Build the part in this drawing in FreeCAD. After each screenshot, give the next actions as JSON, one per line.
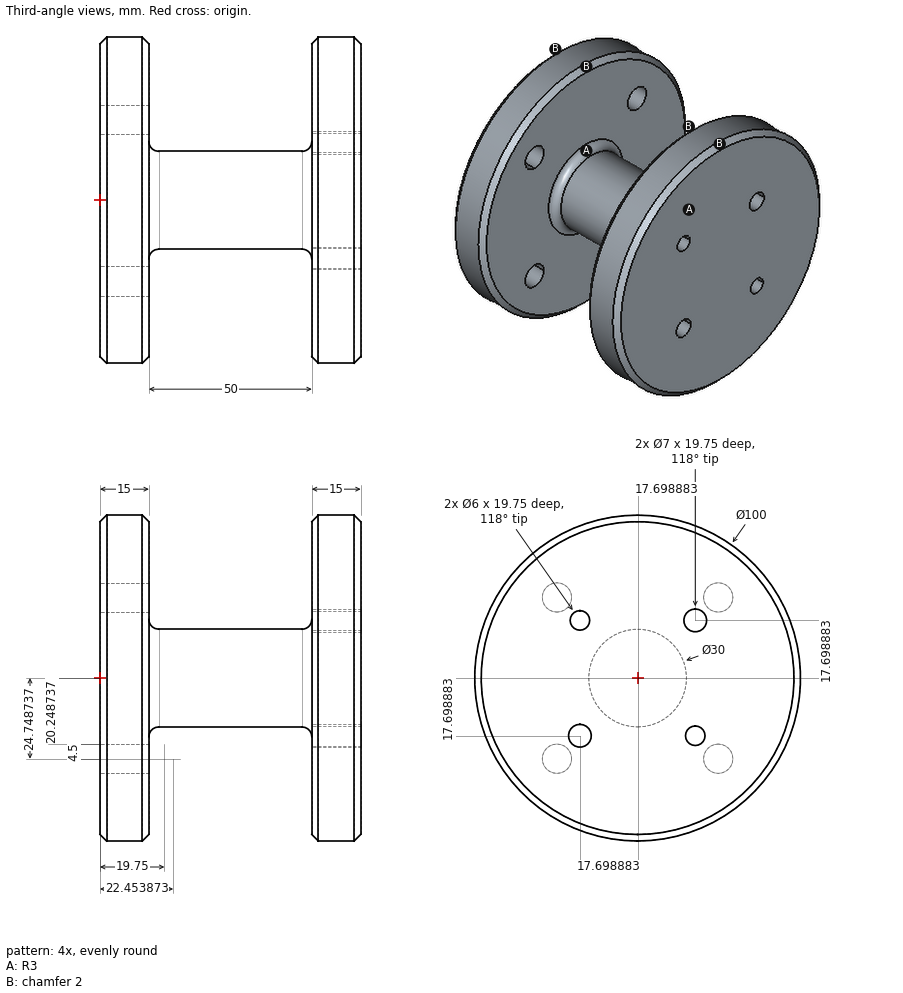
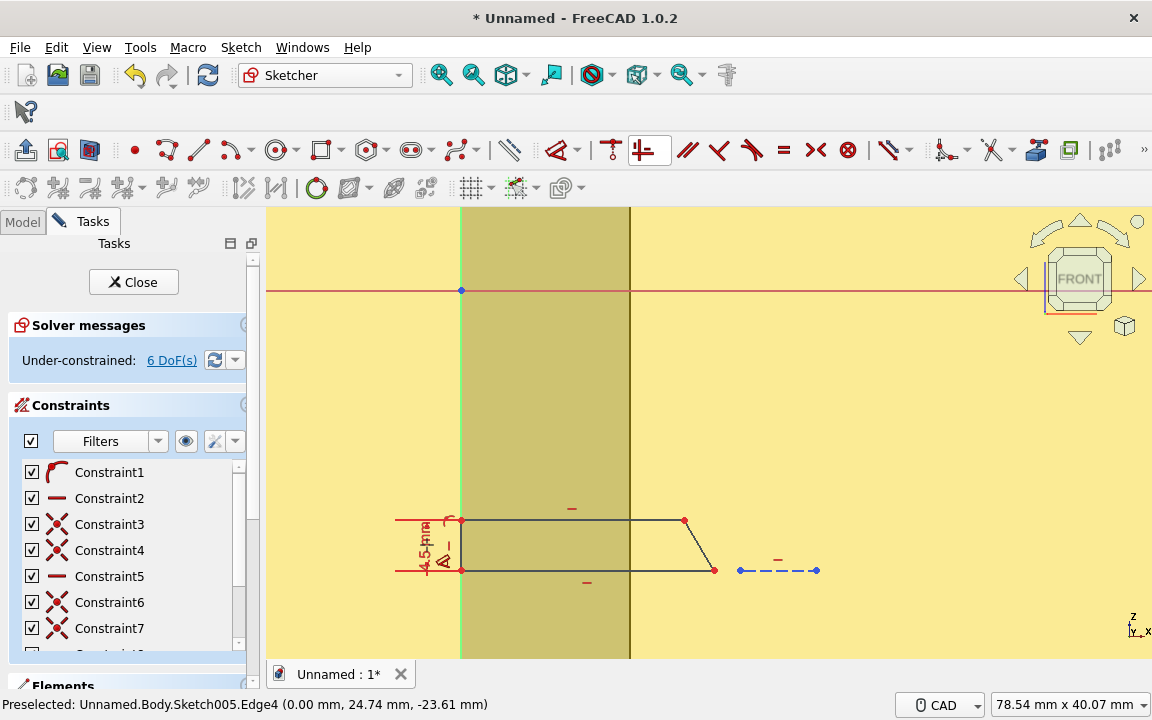
{"action": "left_click", "coordinate": [528, 520]}
{"action": "left_click", "coordinate": [573, 554]}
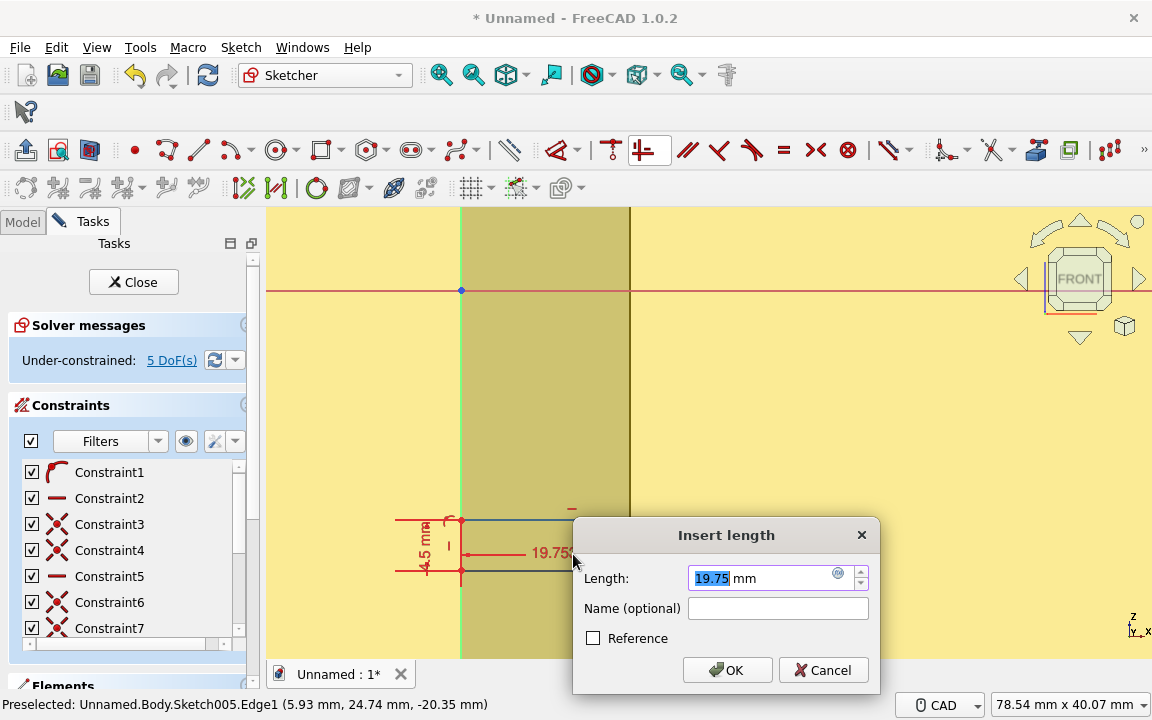
{"action": "type", "text": "19.75"}
{"action": "key", "text": "Return"}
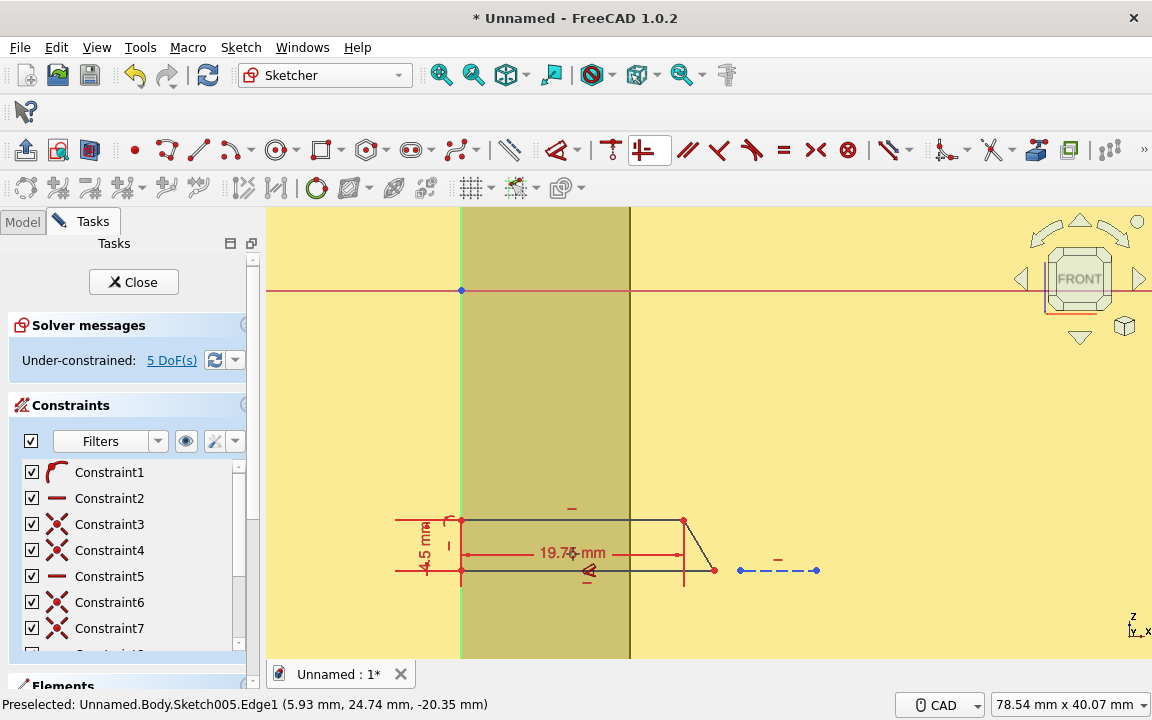
{"action": "left_click", "coordinate": [638, 571]}
{"action": "left_click", "coordinate": [588, 605]}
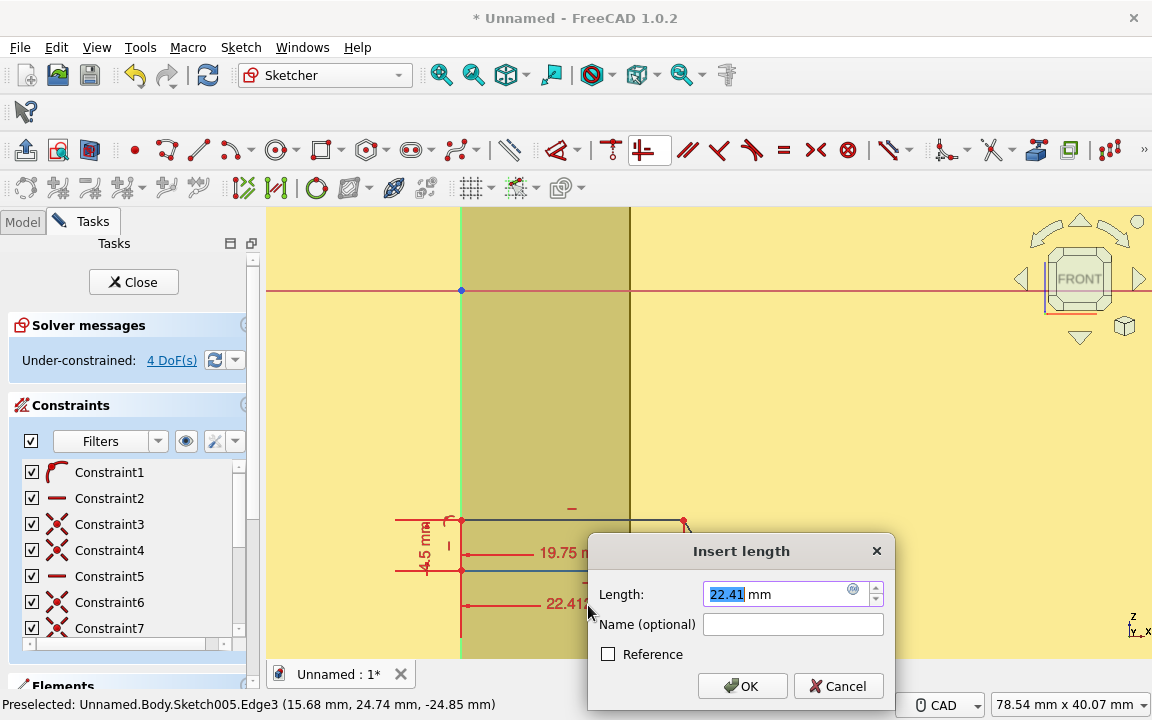
{"action": "type", "text": "22.453873"}
{"action": "key", "text": "Return"}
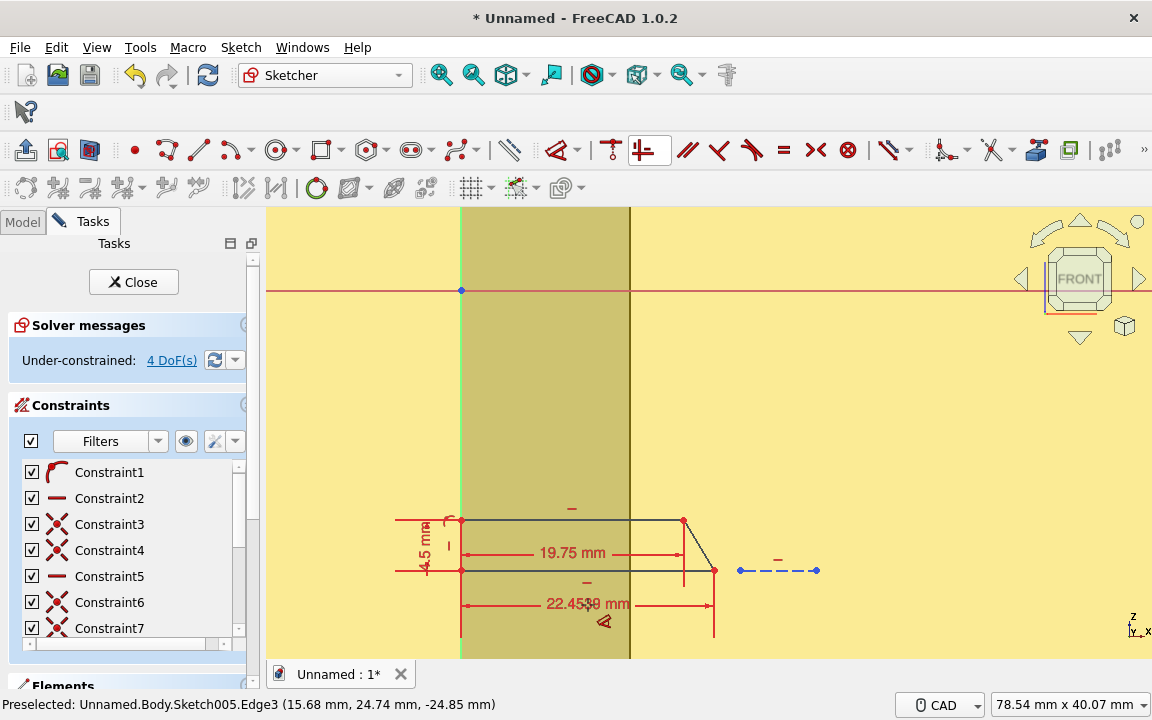
{"action": "left_click", "coordinate": [461, 520]}
{"action": "left_click", "coordinate": [427, 405]}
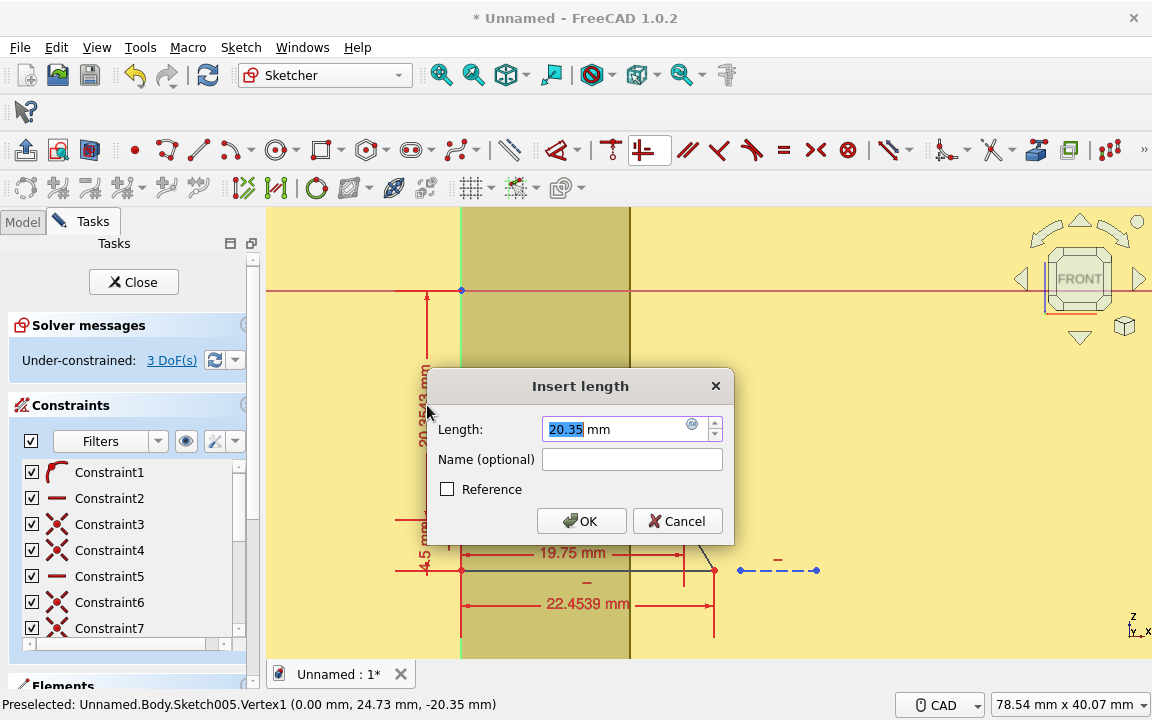
{"action": "type", "text": "20.248737"}
{"action": "key", "text": "Return"}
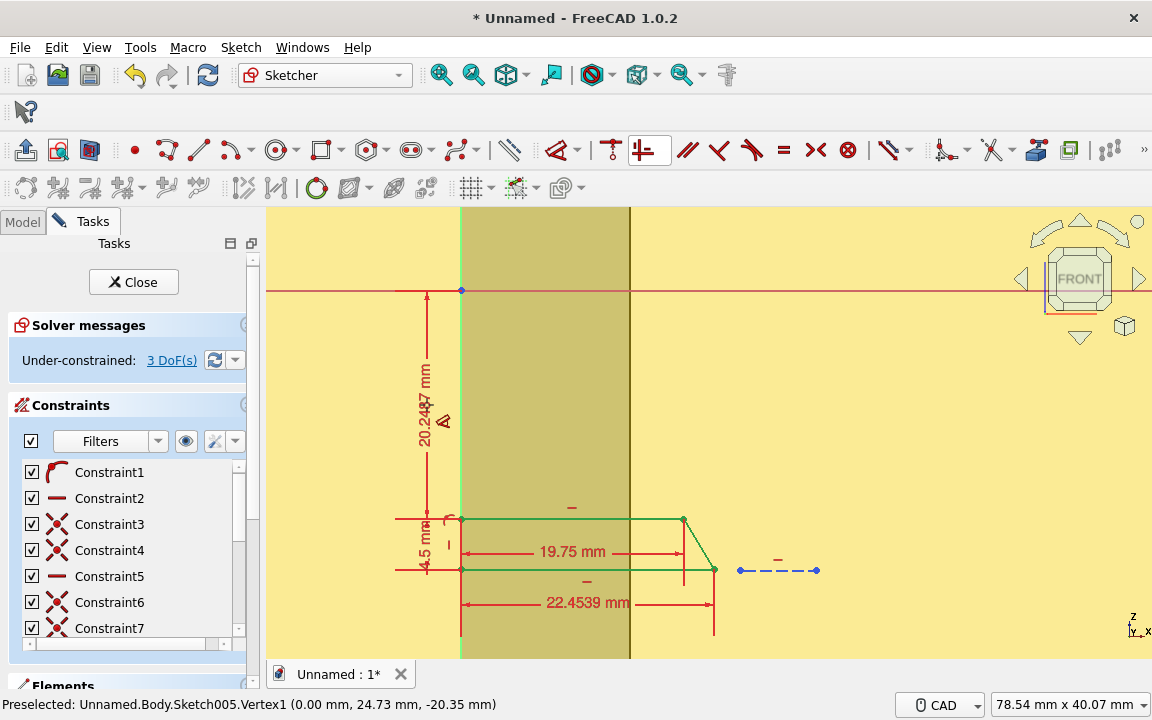
{"action": "left_click", "coordinate": [740, 571]}
{"action": "left_click", "coordinate": [427, 431]}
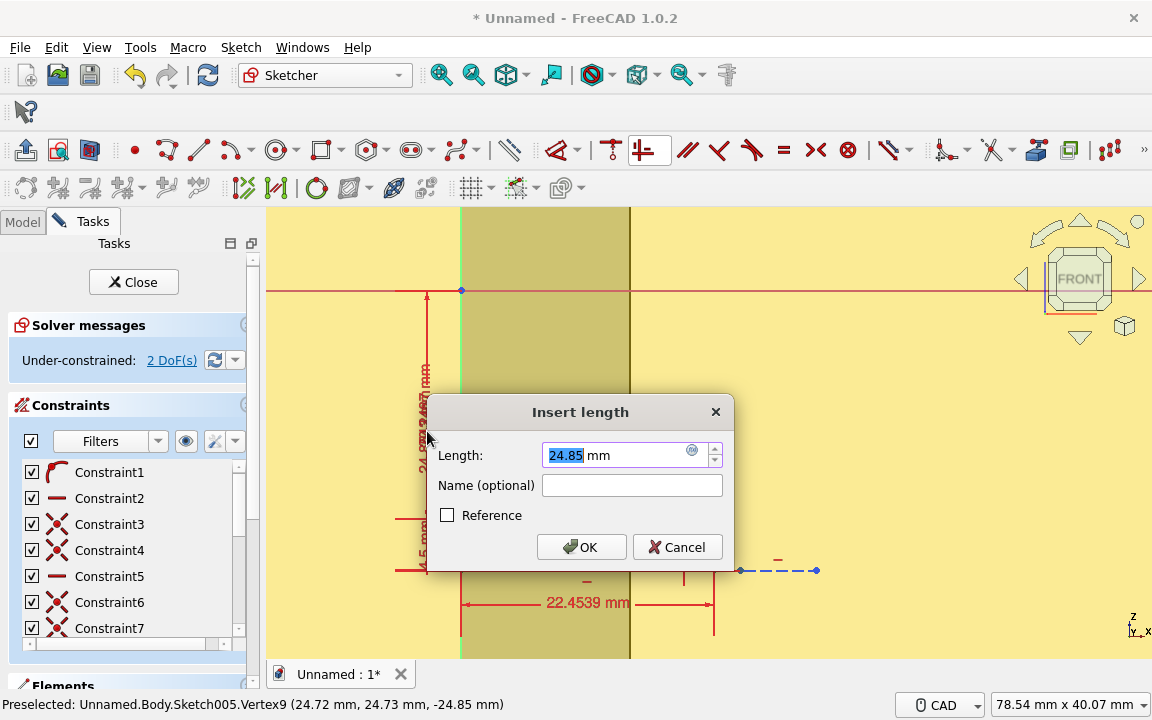
{"action": "type", "text": "24.748737"}
{"action": "key", "text": "Return"}
{"action": "key", "text": "Escape"}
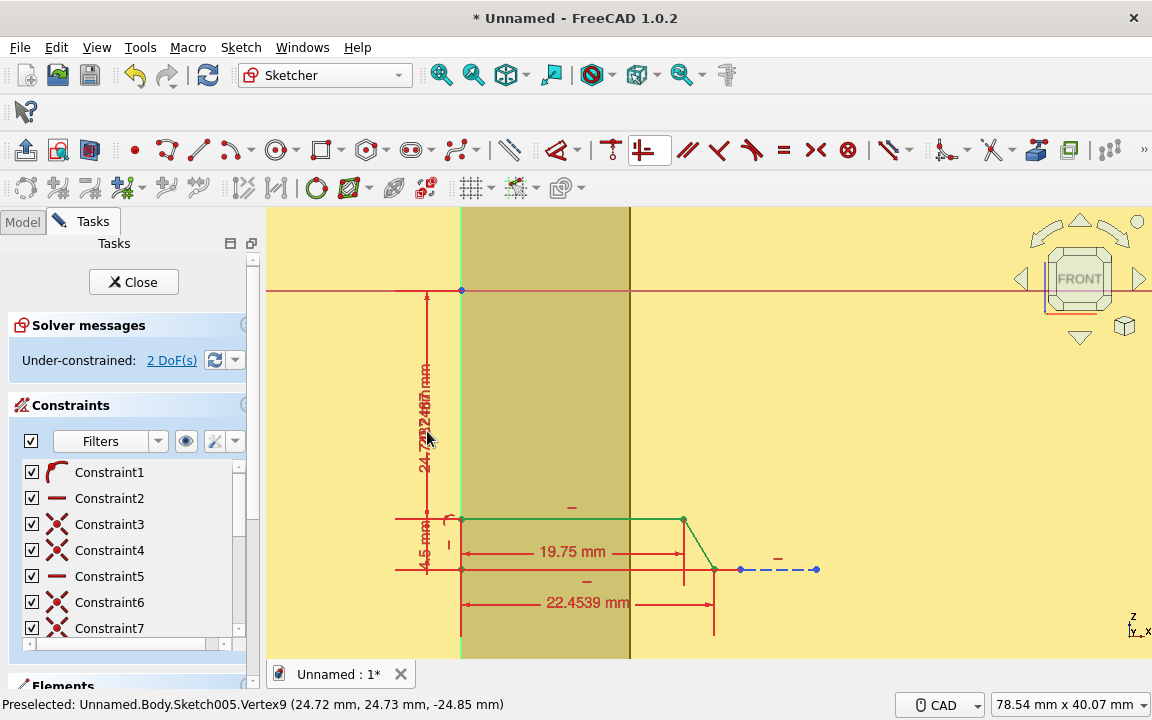
{"action": "left_click", "coordinate": [134, 282]}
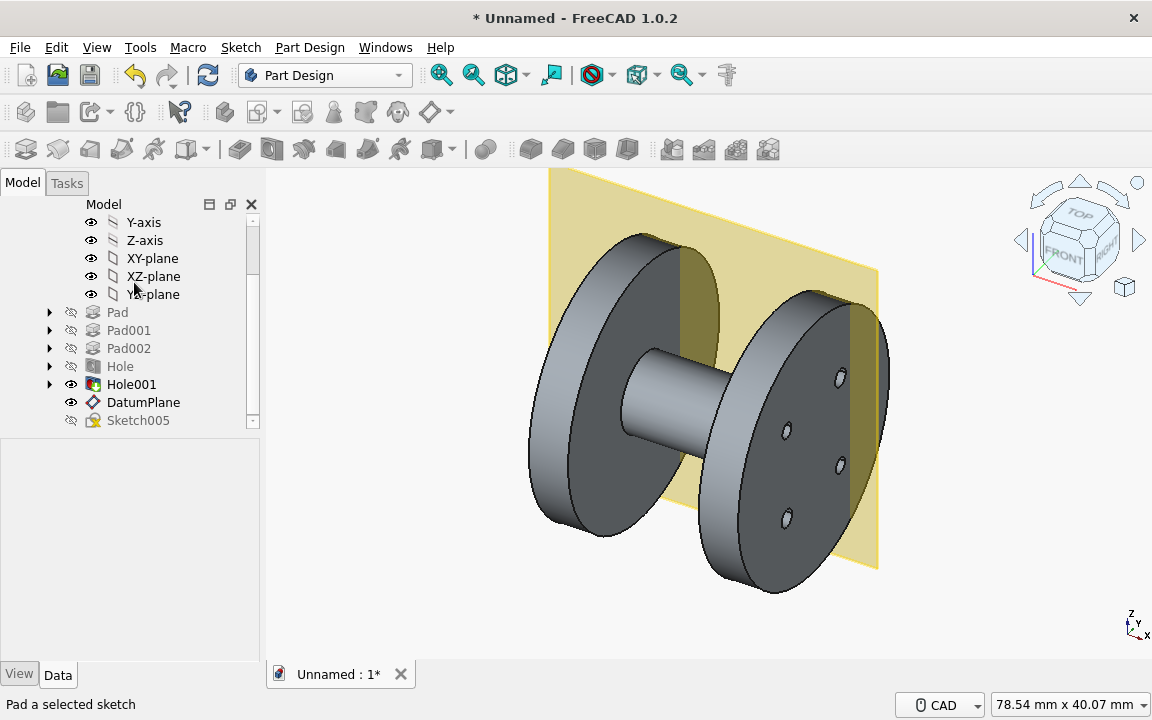
{"action": "left_click", "coordinate": [304, 150]}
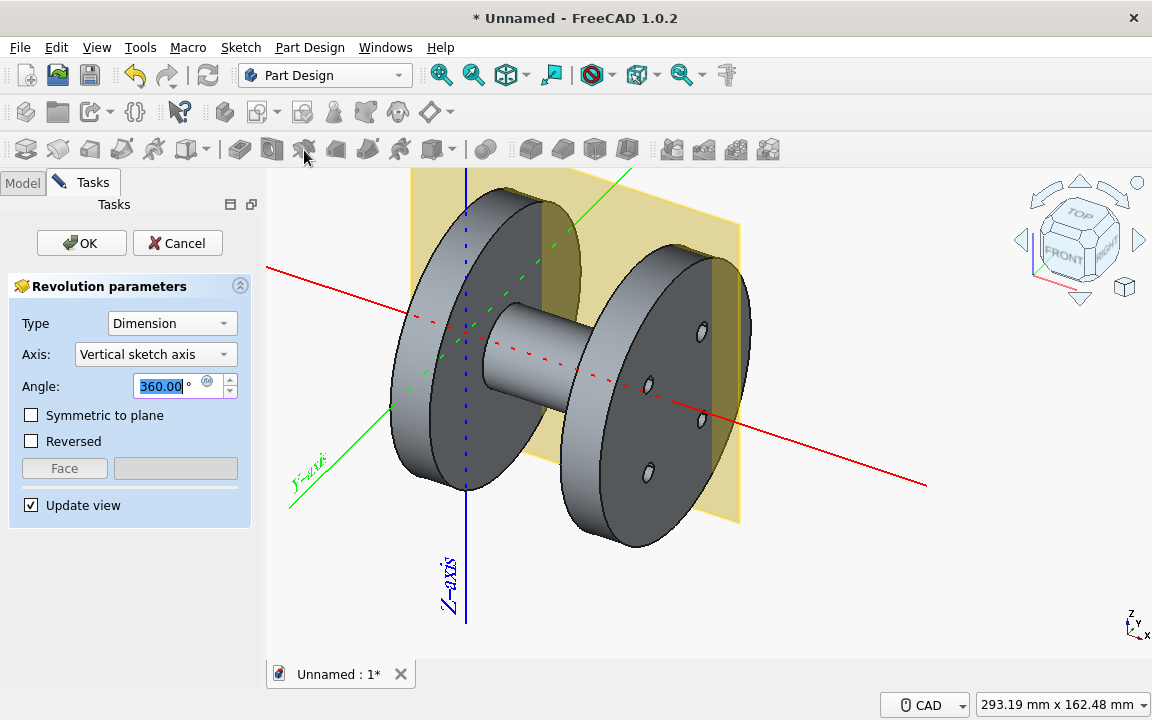
{"action": "left_click", "coordinate": [156, 354]}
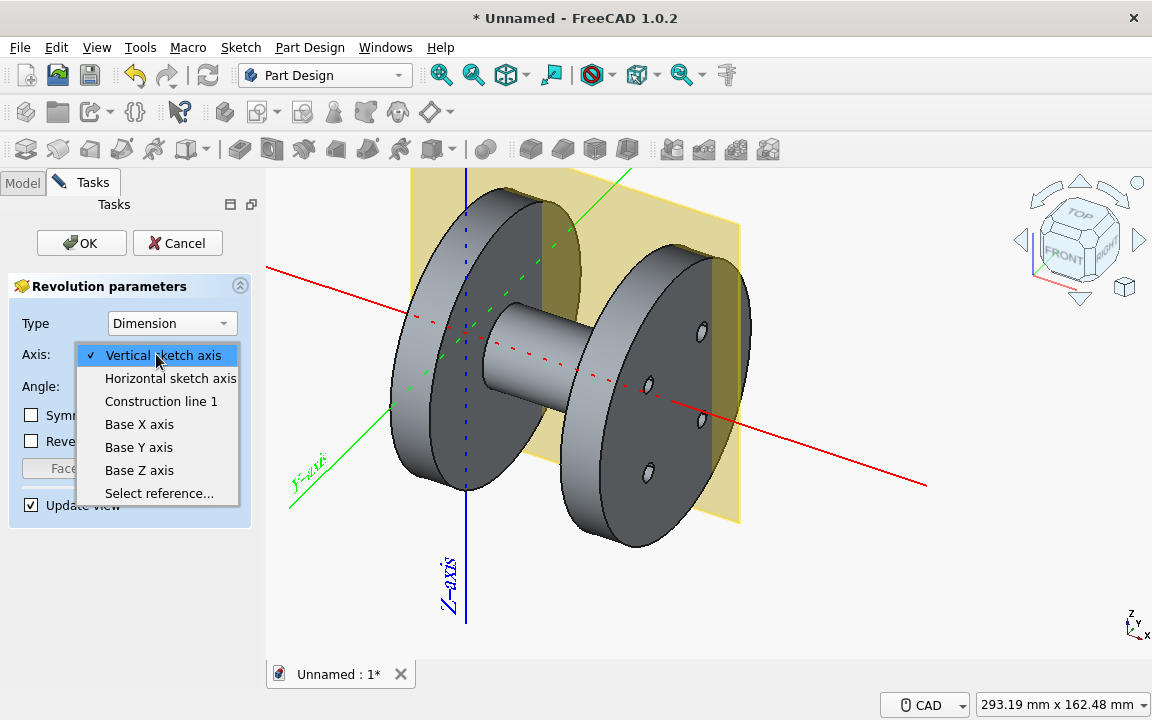
{"action": "left_click", "coordinate": [156, 402]}